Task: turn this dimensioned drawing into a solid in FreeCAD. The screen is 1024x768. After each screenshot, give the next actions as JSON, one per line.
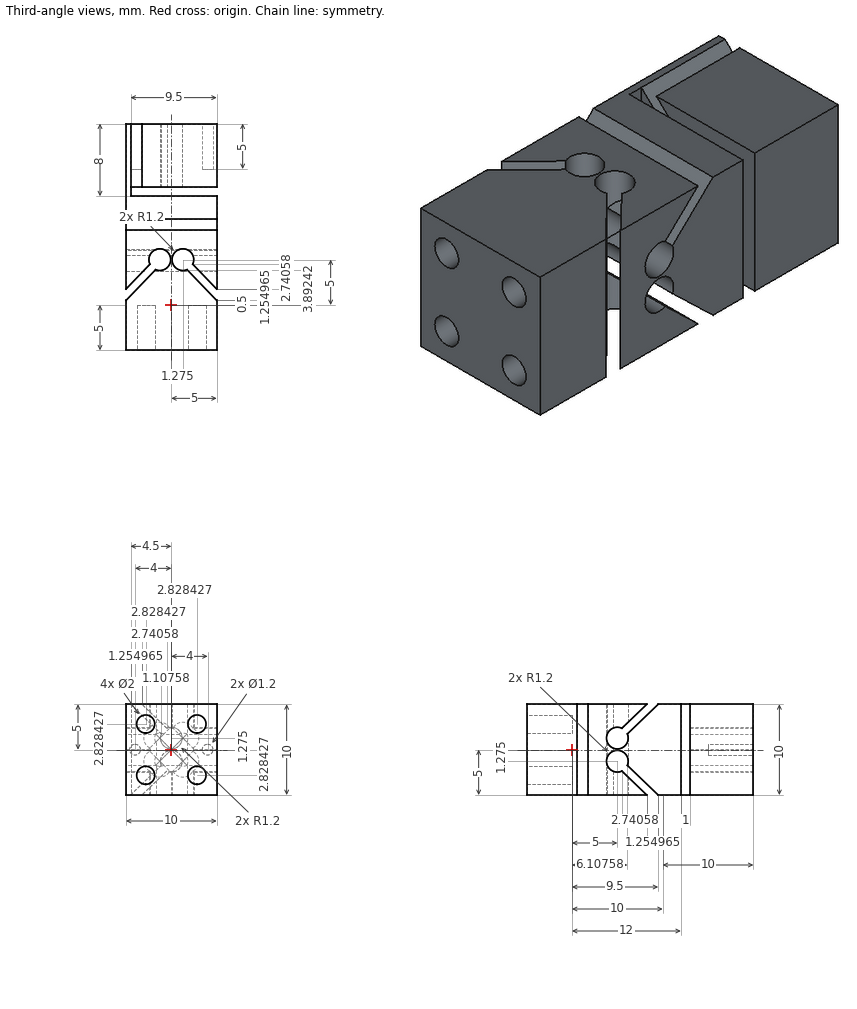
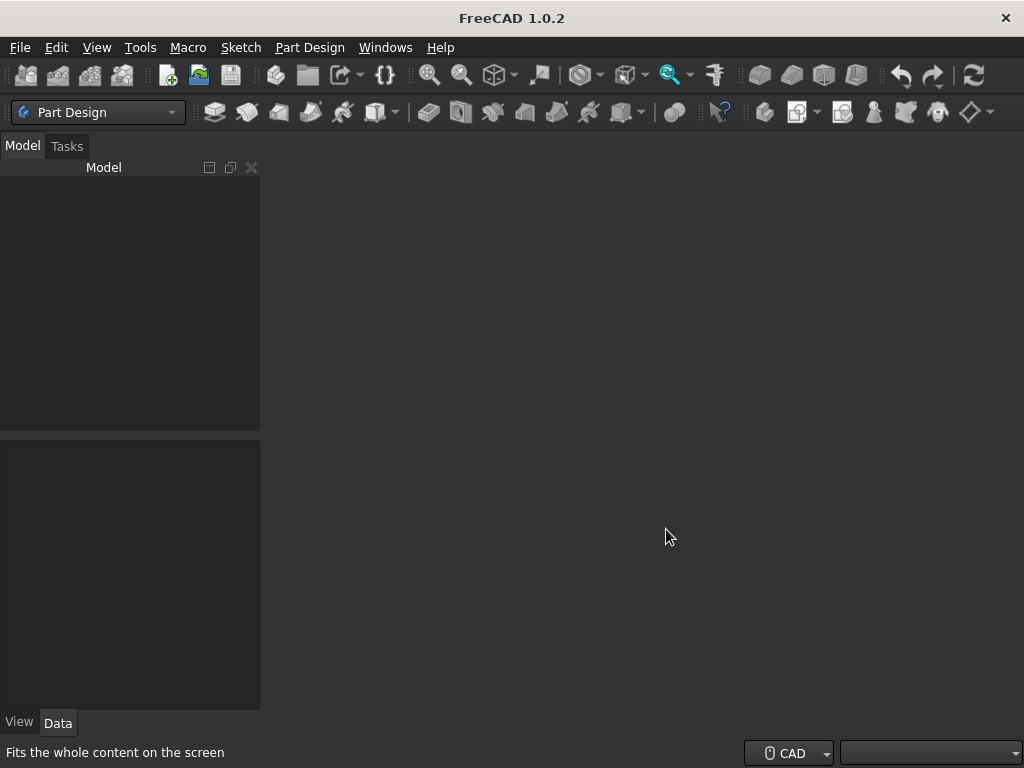
{"action": "left_click", "coordinate": [168, 76]}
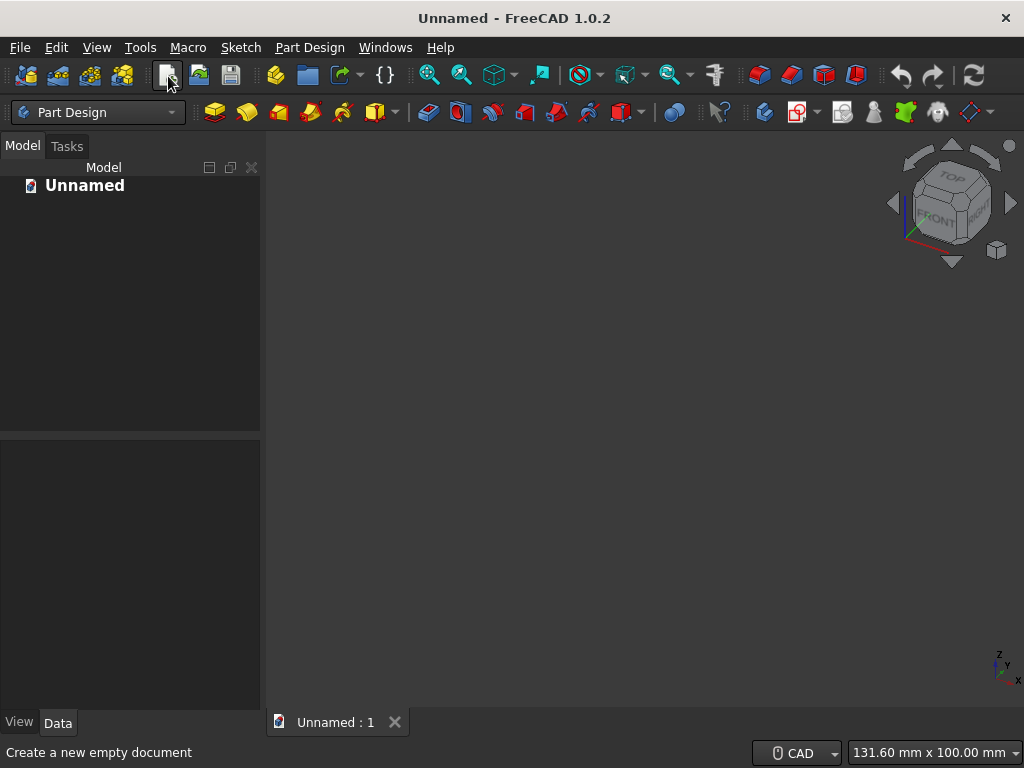
{"action": "left_click", "coordinate": [798, 112]}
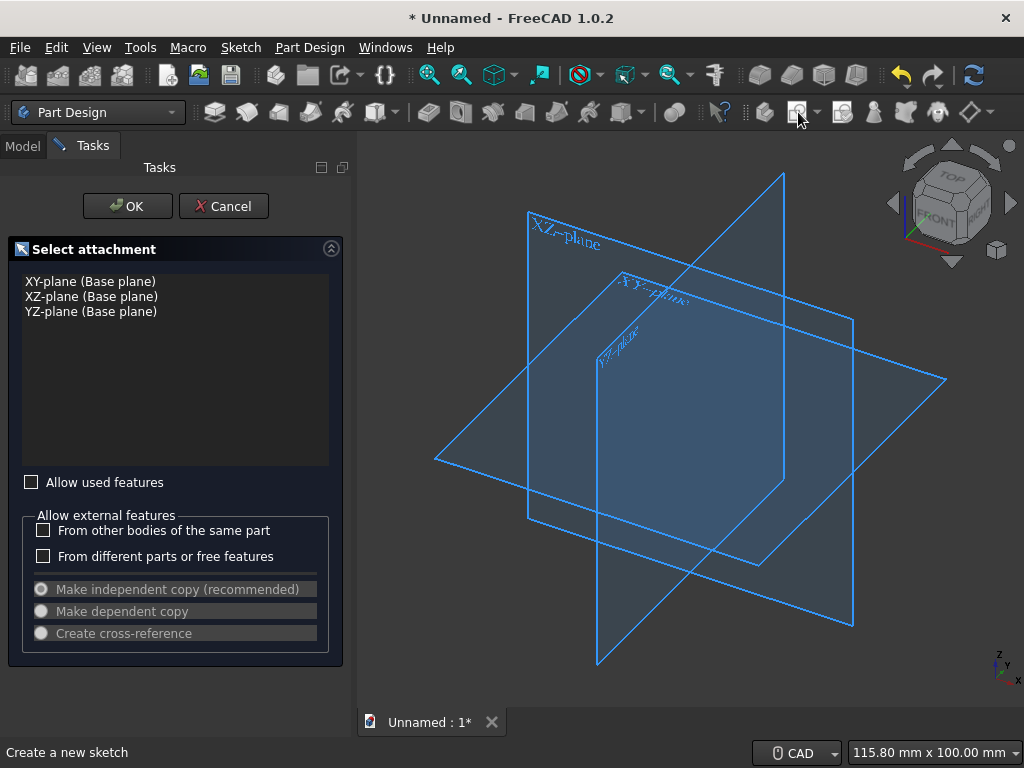
{"action": "left_click", "coordinate": [82, 296]}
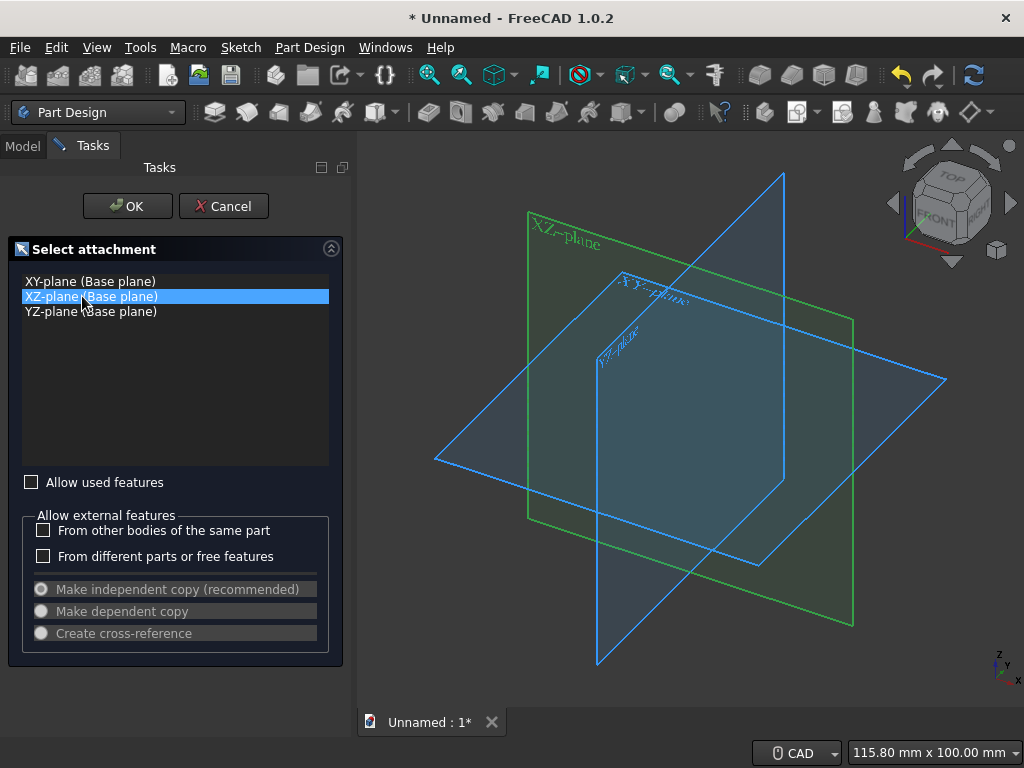
{"action": "left_click", "coordinate": [128, 206]}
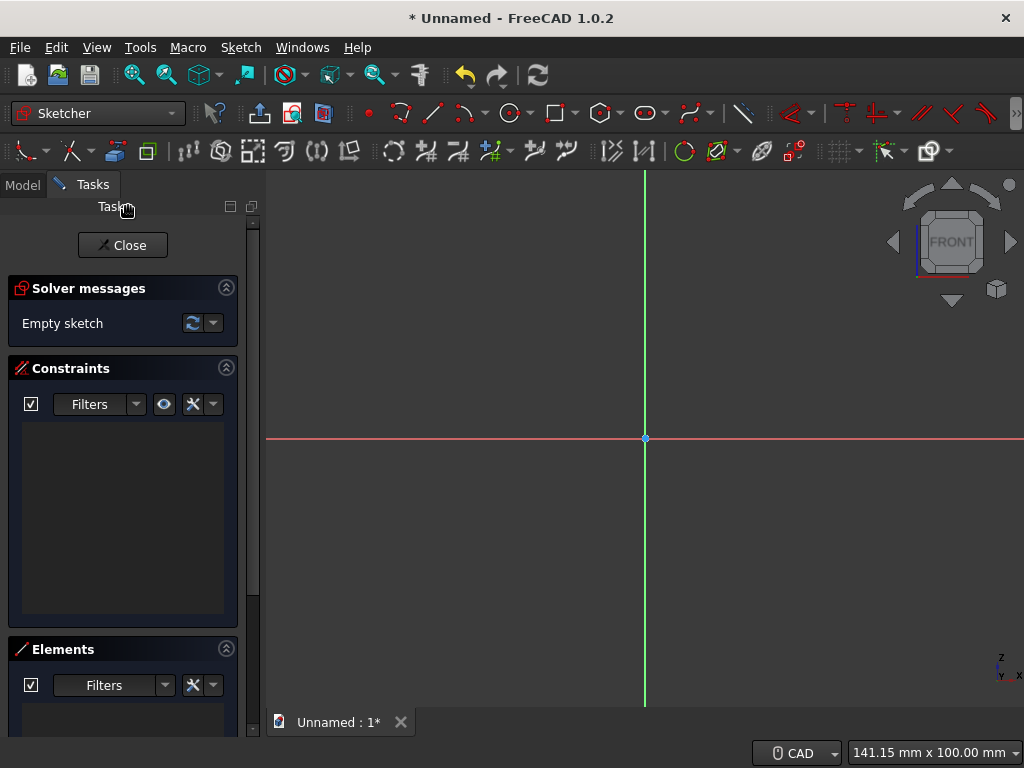
{"action": "scroll", "coordinate": [659, 438], "scroll_direction": "up", "scroll_amount": 9}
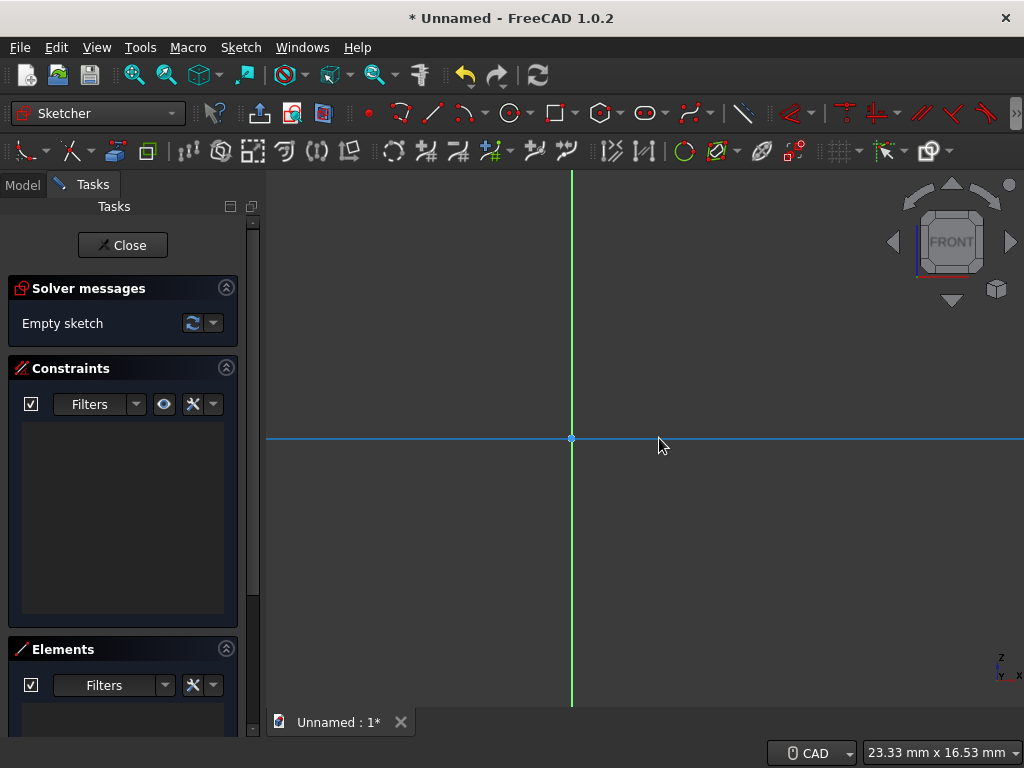
{"action": "left_click", "coordinate": [578, 114]}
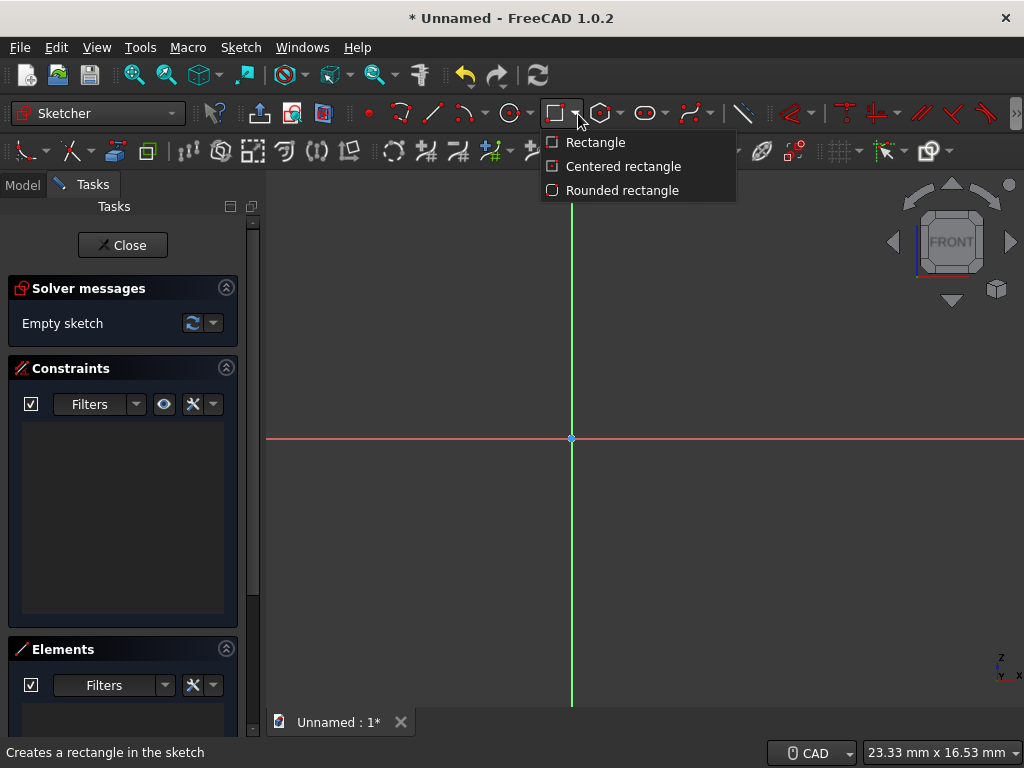
{"action": "left_click", "coordinate": [638, 166]}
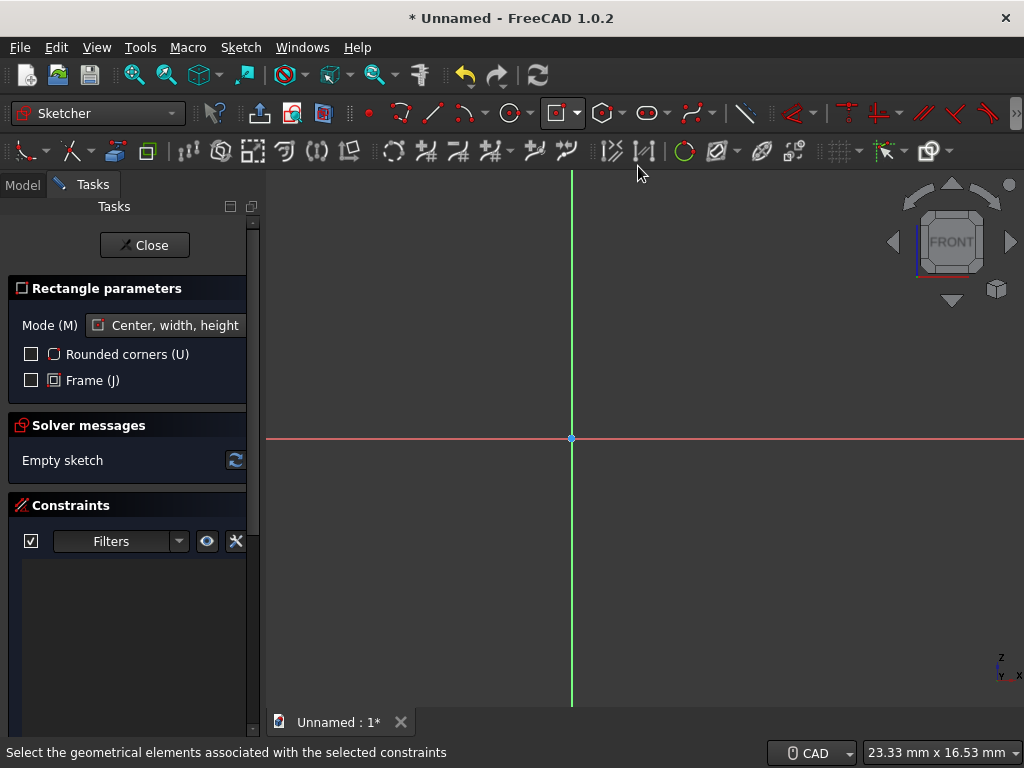
{"action": "left_click", "coordinate": [572, 438]}
{"action": "left_click", "coordinate": [734, 276]}
{"action": "key", "text": "Escape"}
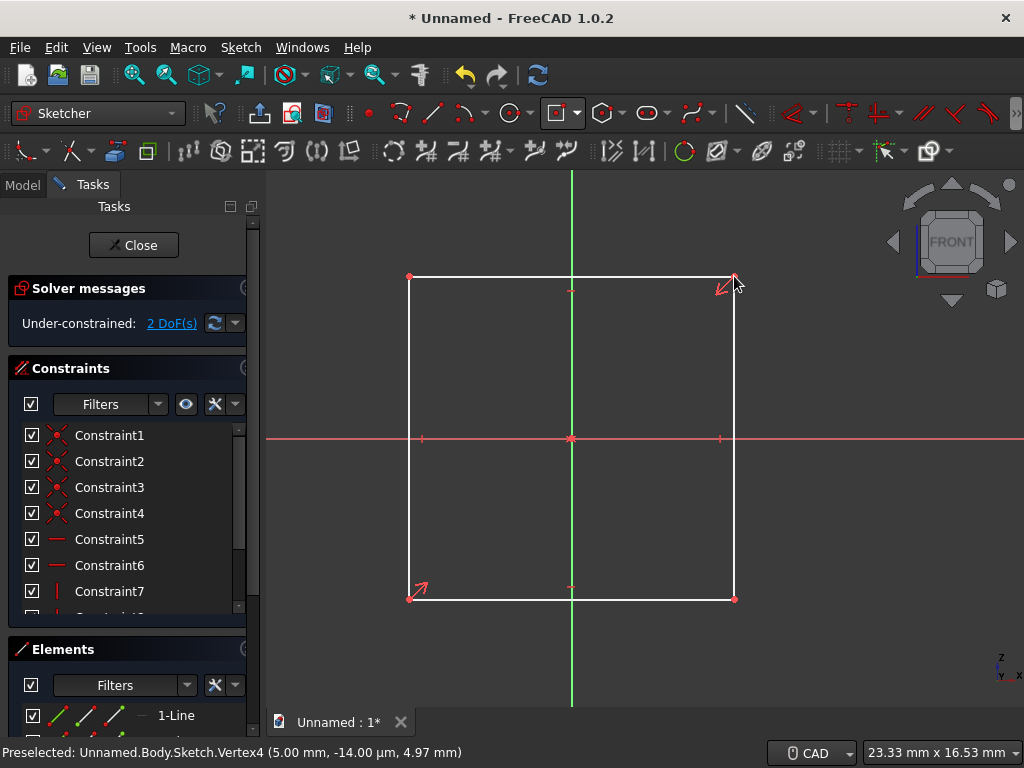
{"action": "left_click", "coordinate": [507, 600]}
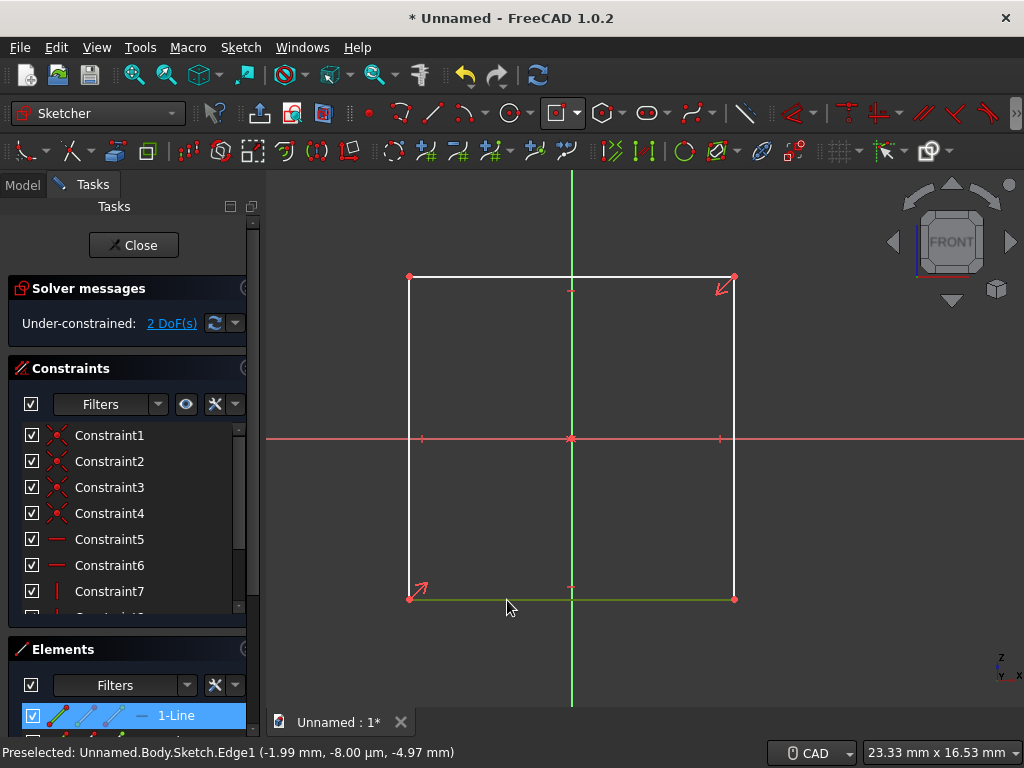
{"action": "key", "text": "l"}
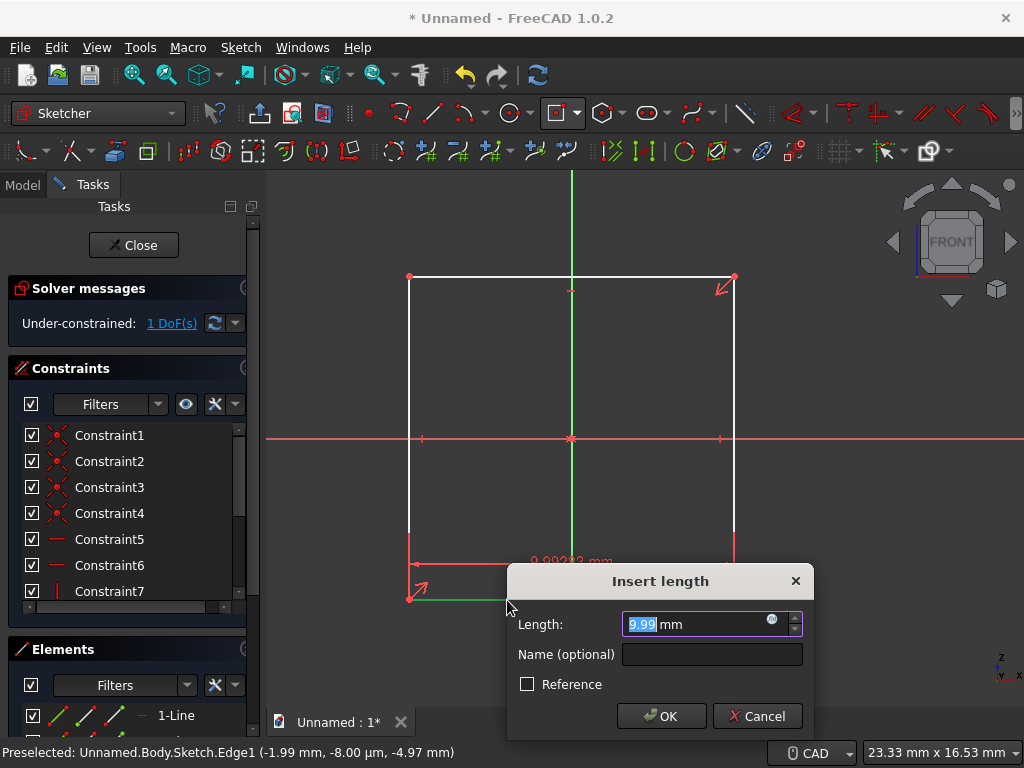
{"action": "type", "text": "10"}
{"action": "key", "text": "Return"}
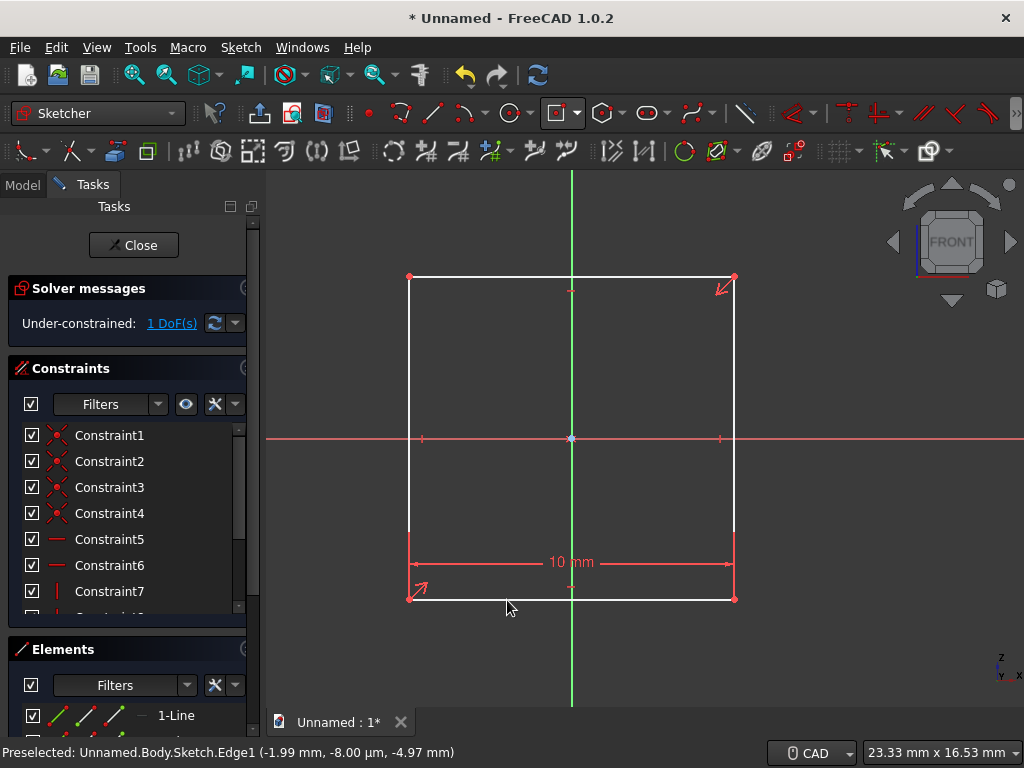
{"action": "left_click", "coordinate": [734, 503]}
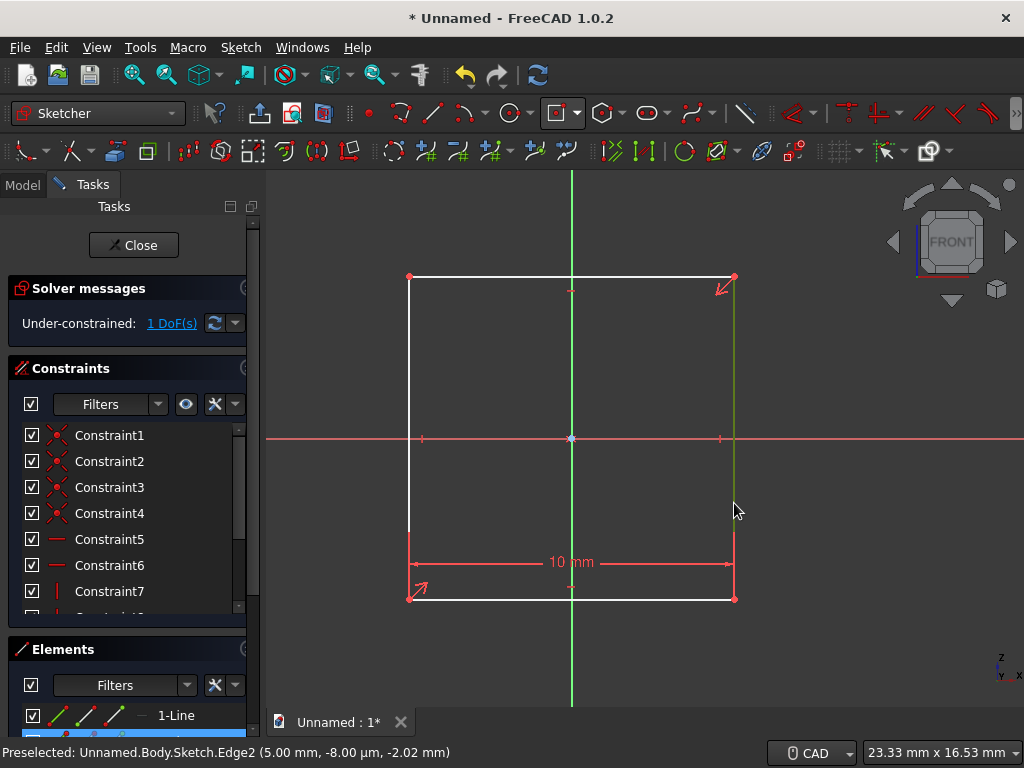
{"action": "left_click", "coordinate": [816, 114]}